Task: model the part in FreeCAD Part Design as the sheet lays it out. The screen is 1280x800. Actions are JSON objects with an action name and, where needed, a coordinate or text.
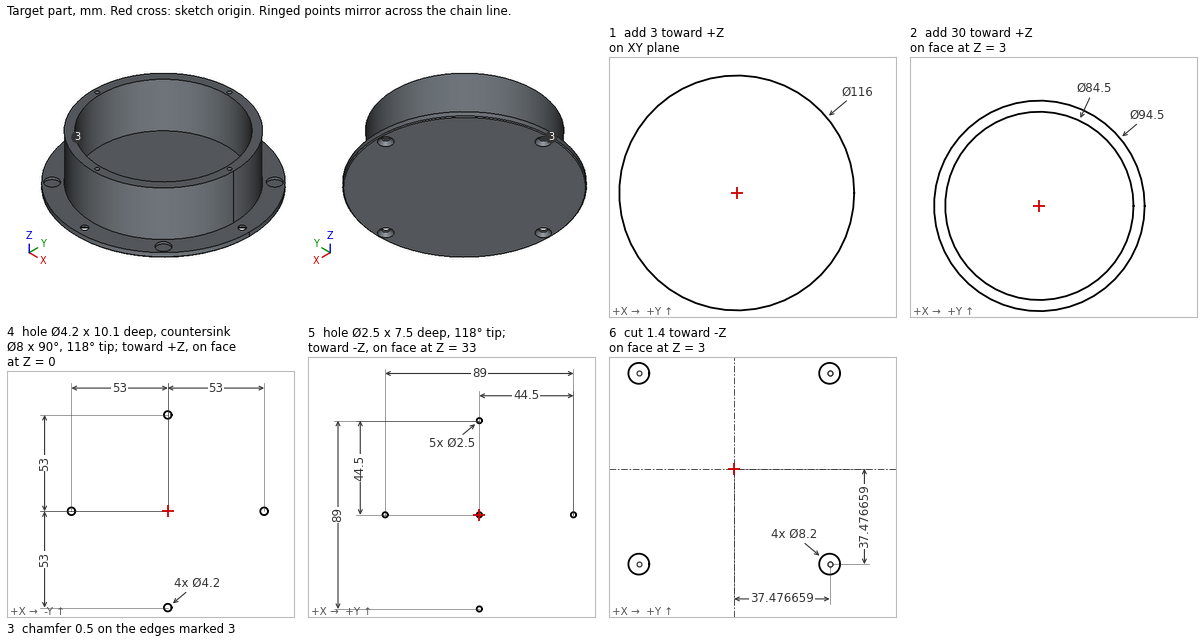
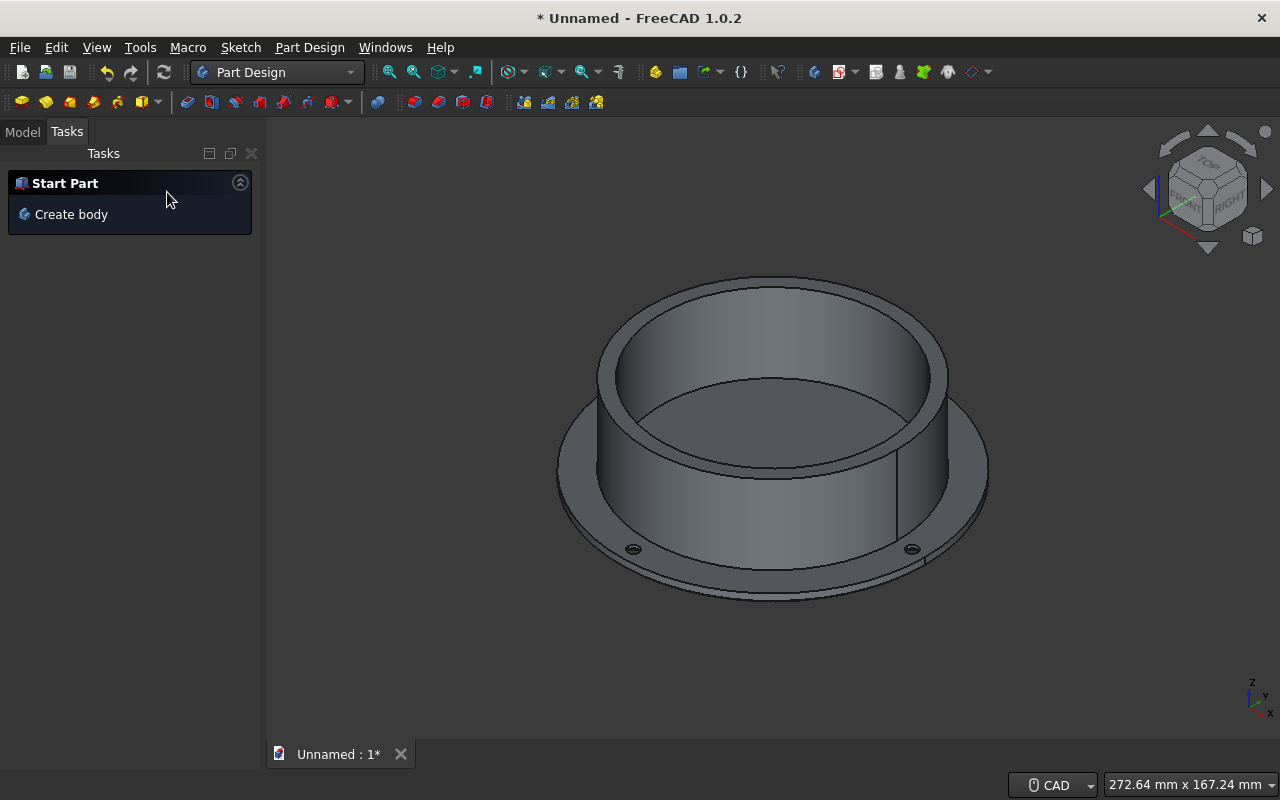
{"action": "scroll", "coordinate": [915, 418], "scroll_direction": "up", "scroll_amount": 10}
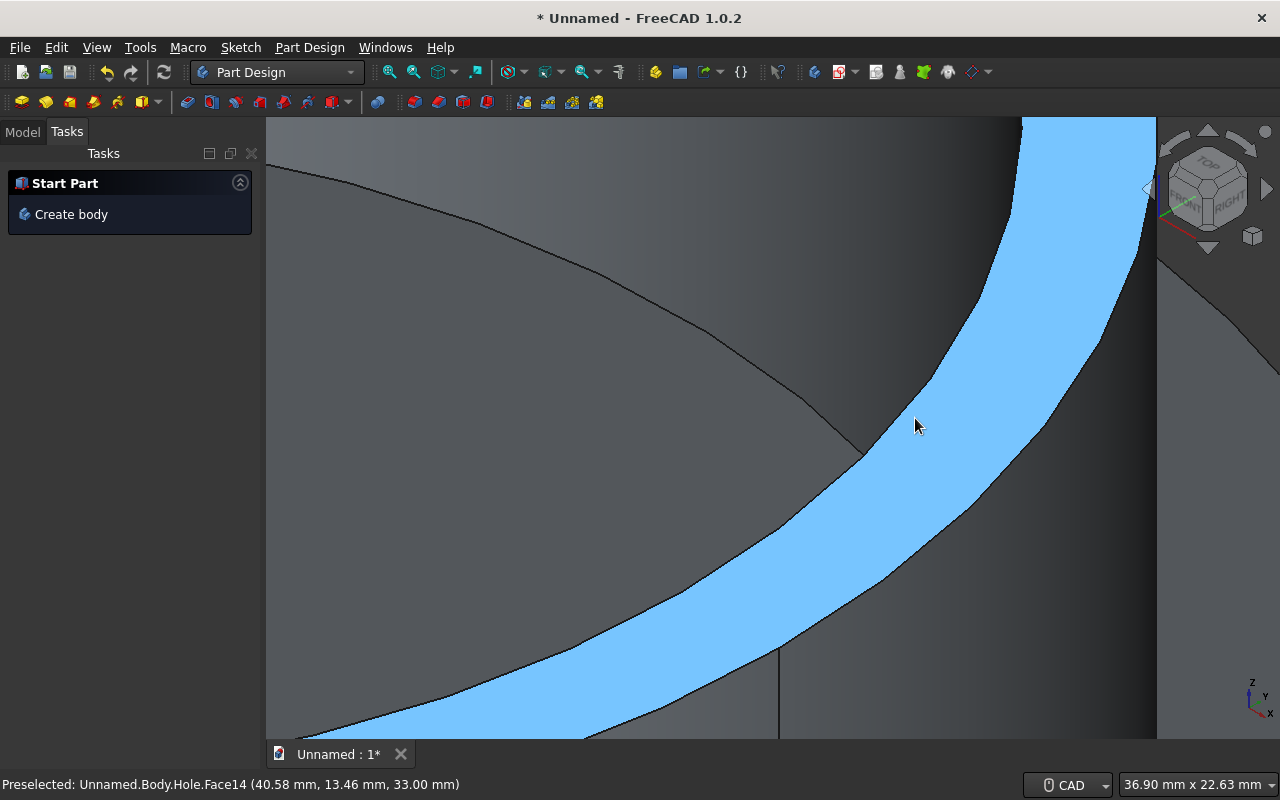
{"action": "left_click", "coordinate": [910, 420]}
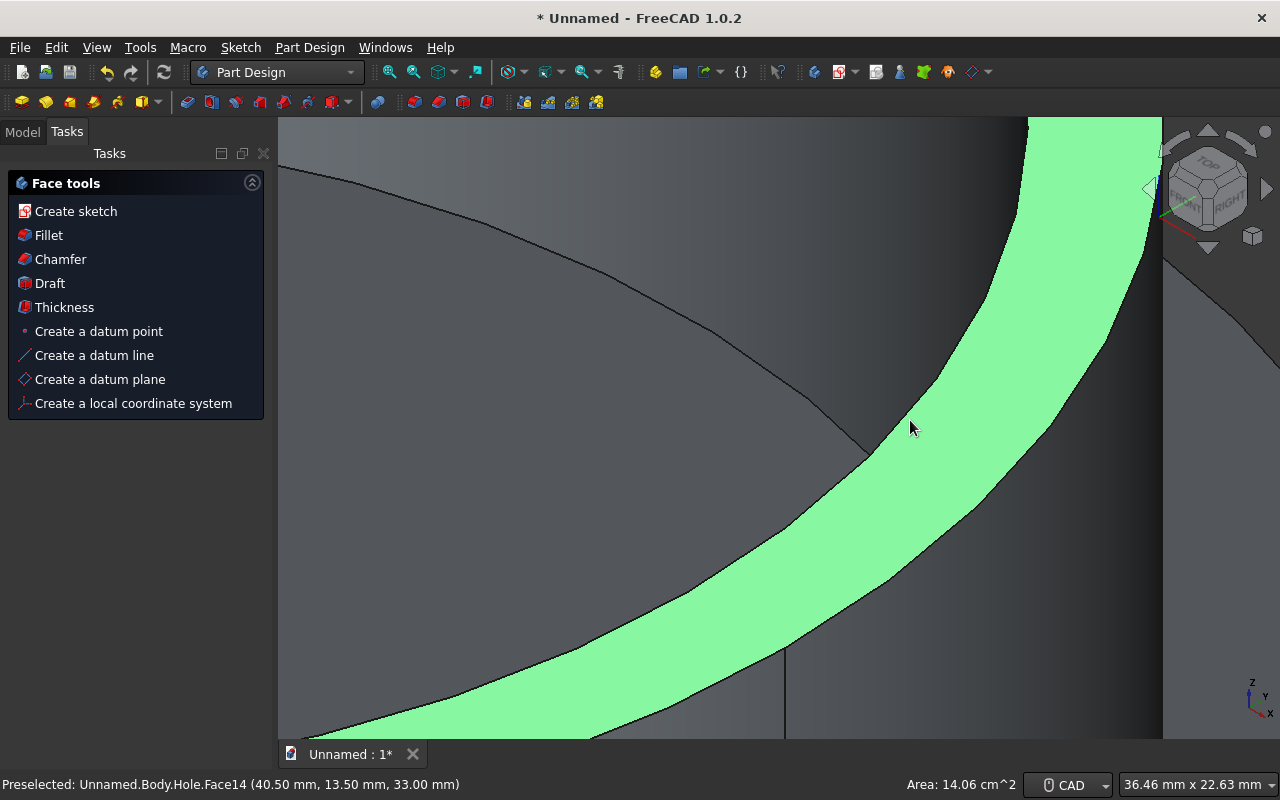
{"action": "left_click", "coordinate": [840, 72]}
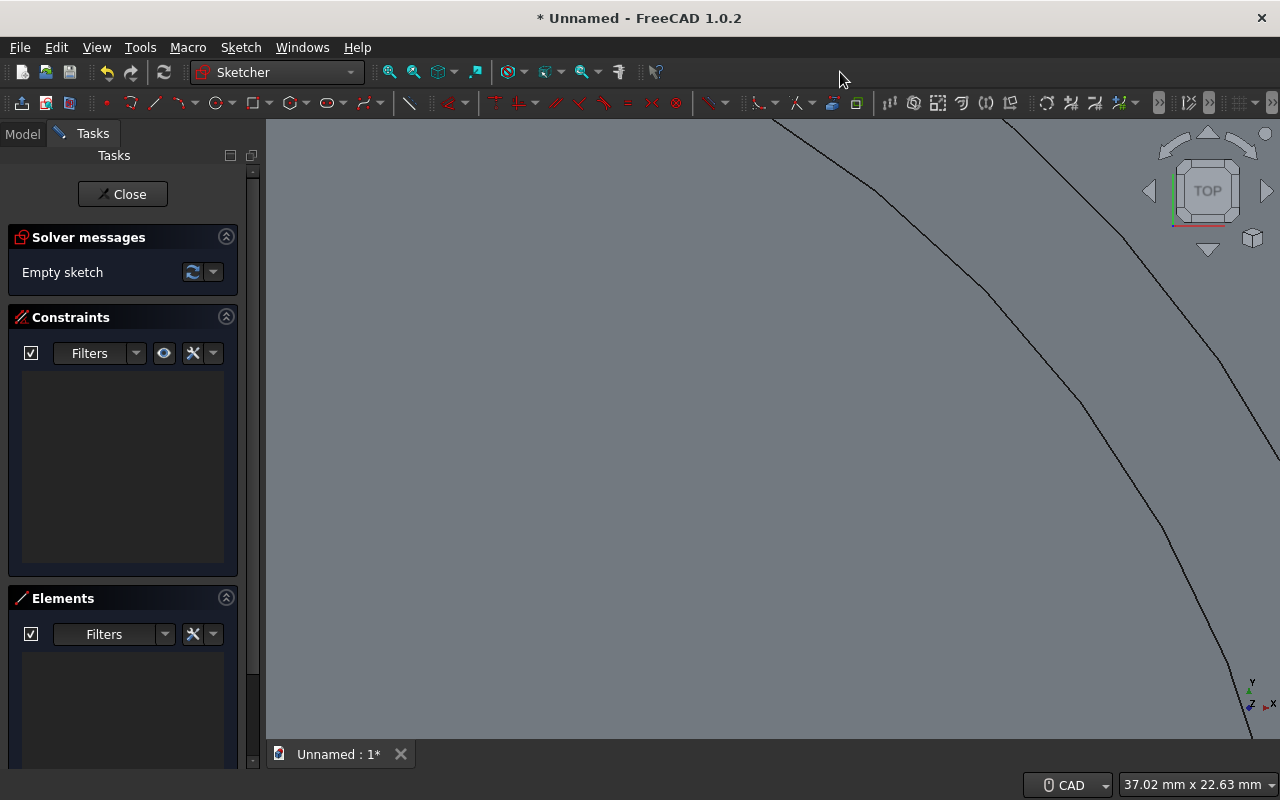
{"action": "scroll", "coordinate": [813, 297], "scroll_direction": "down", "scroll_amount": 9}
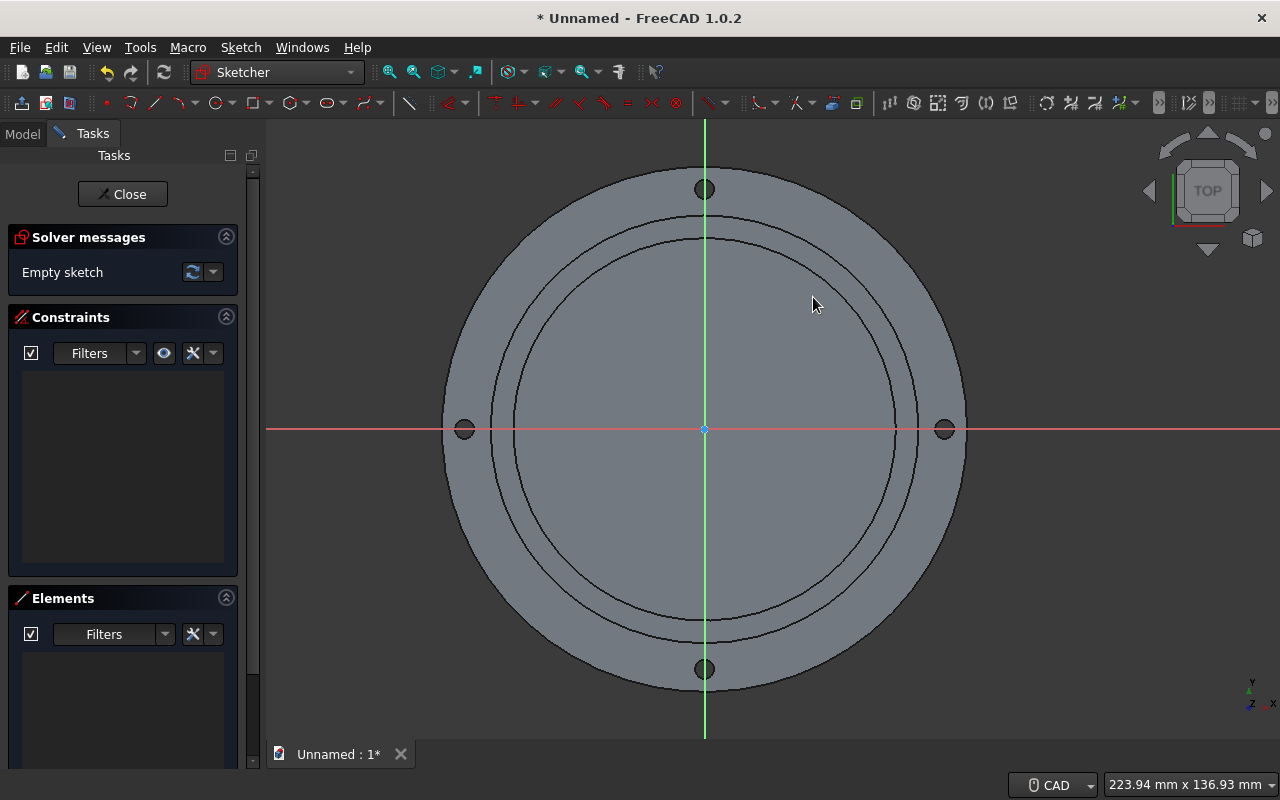
{"action": "left_click", "coordinate": [216, 104]}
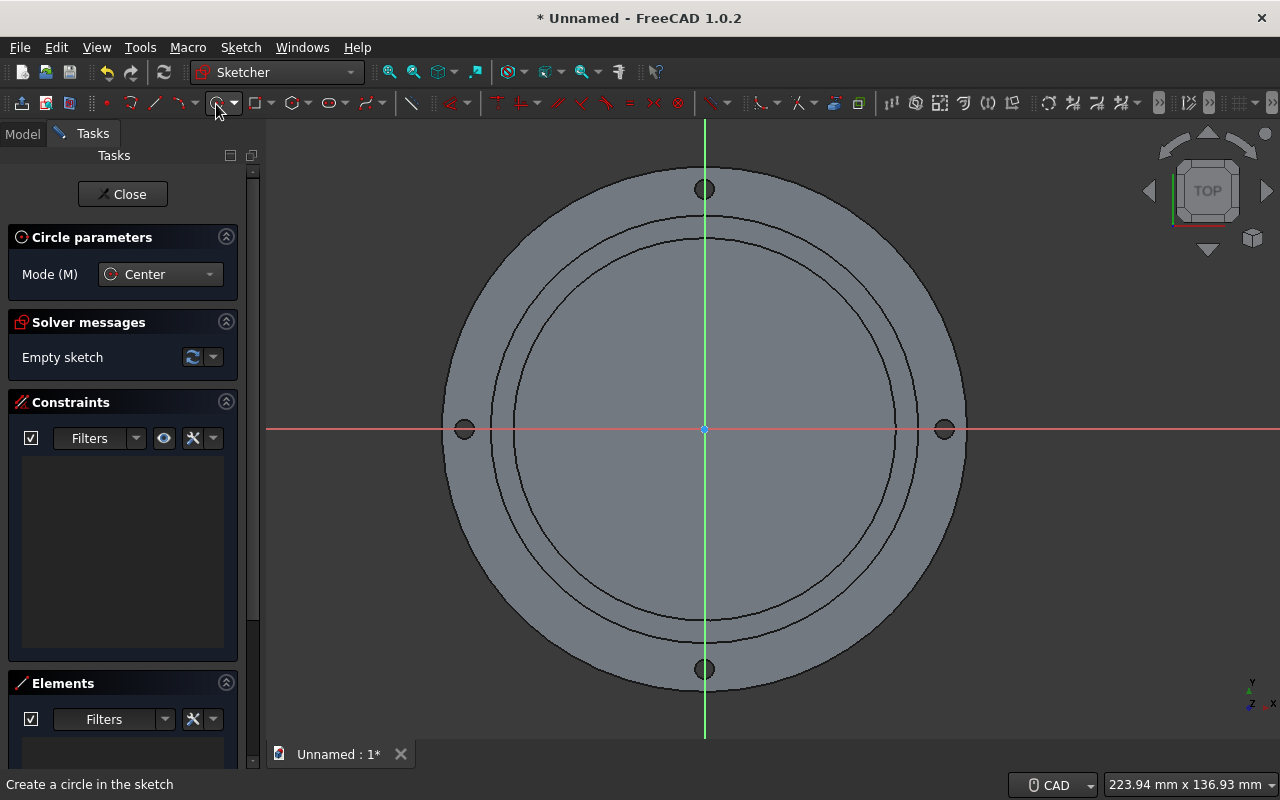
{"action": "scroll", "coordinate": [705, 228], "scroll_direction": "up", "scroll_amount": 7}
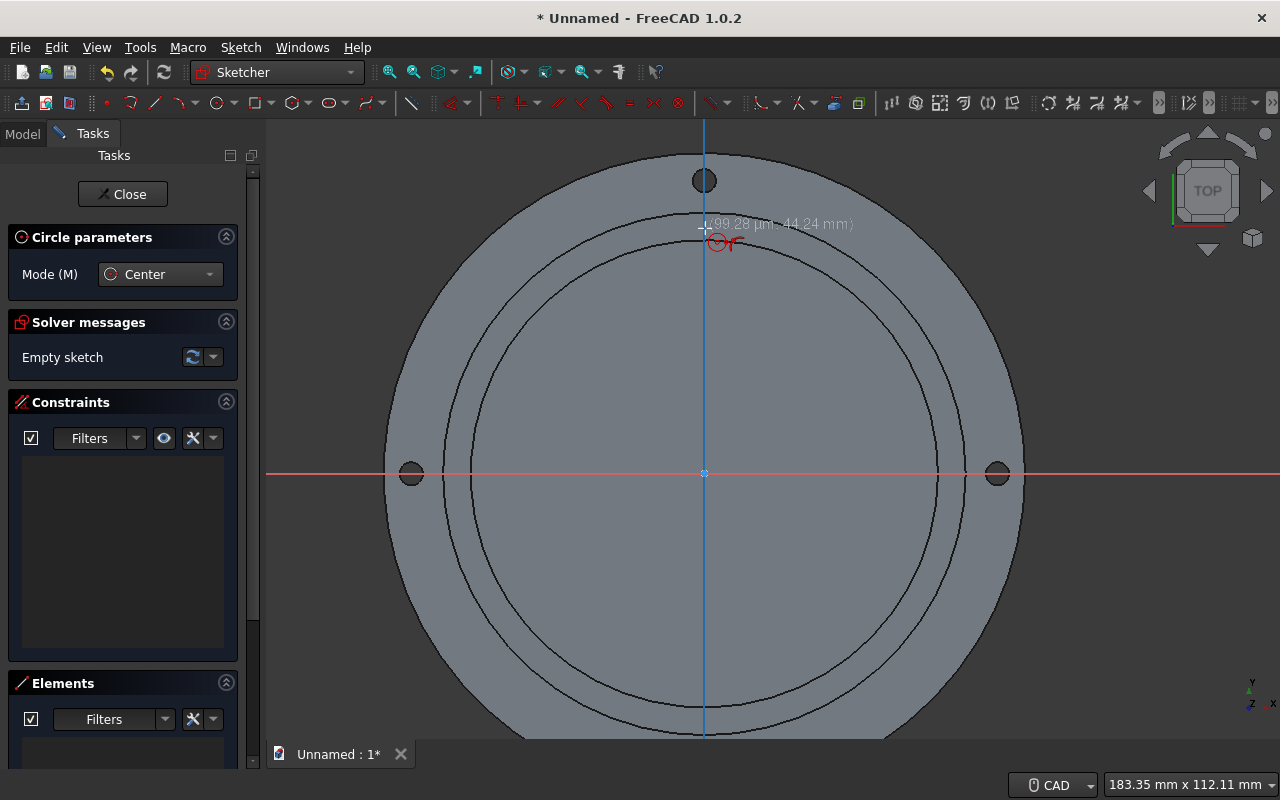
{"action": "scroll", "coordinate": [705, 228], "scroll_direction": "down", "scroll_amount": 7}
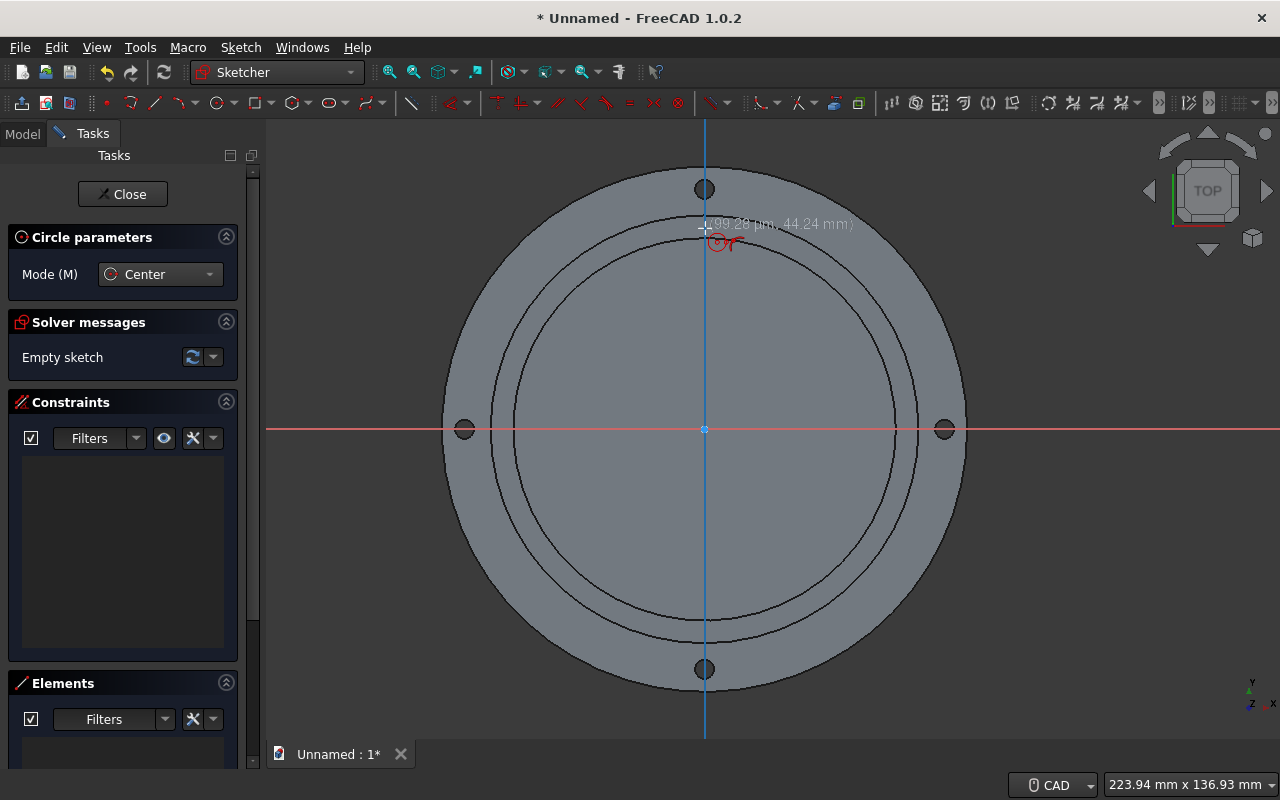
{"action": "left_click", "coordinate": [705, 228]}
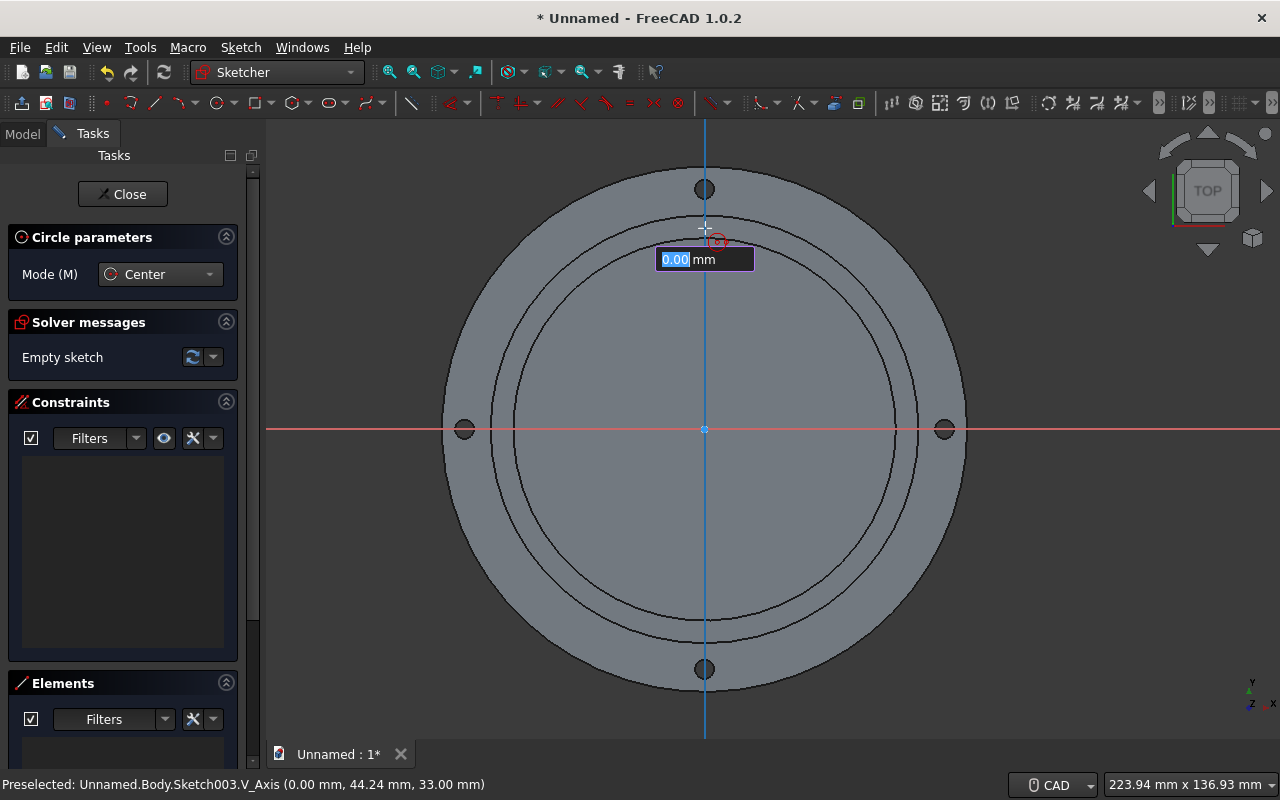
{"action": "scroll", "coordinate": [710, 226], "scroll_direction": "up", "scroll_amount": 6}
{"action": "mouse_move", "coordinate": [709, 225]}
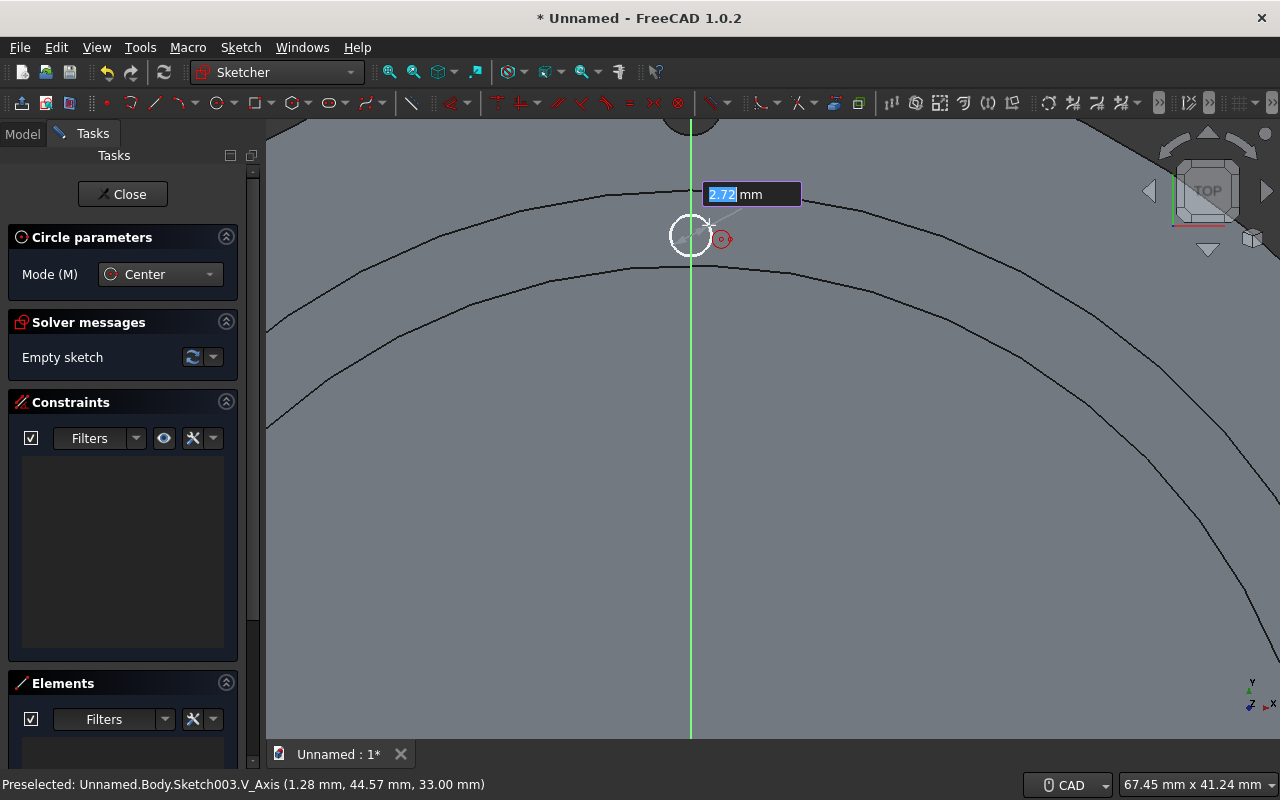
{"action": "type", "text": "2.5"}
{"action": "key", "text": "Return"}